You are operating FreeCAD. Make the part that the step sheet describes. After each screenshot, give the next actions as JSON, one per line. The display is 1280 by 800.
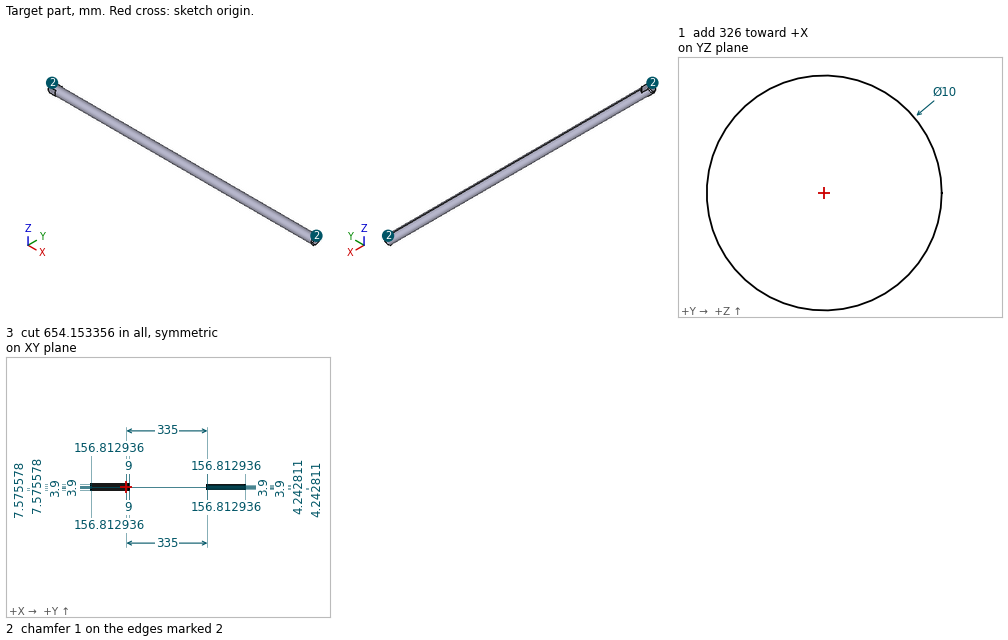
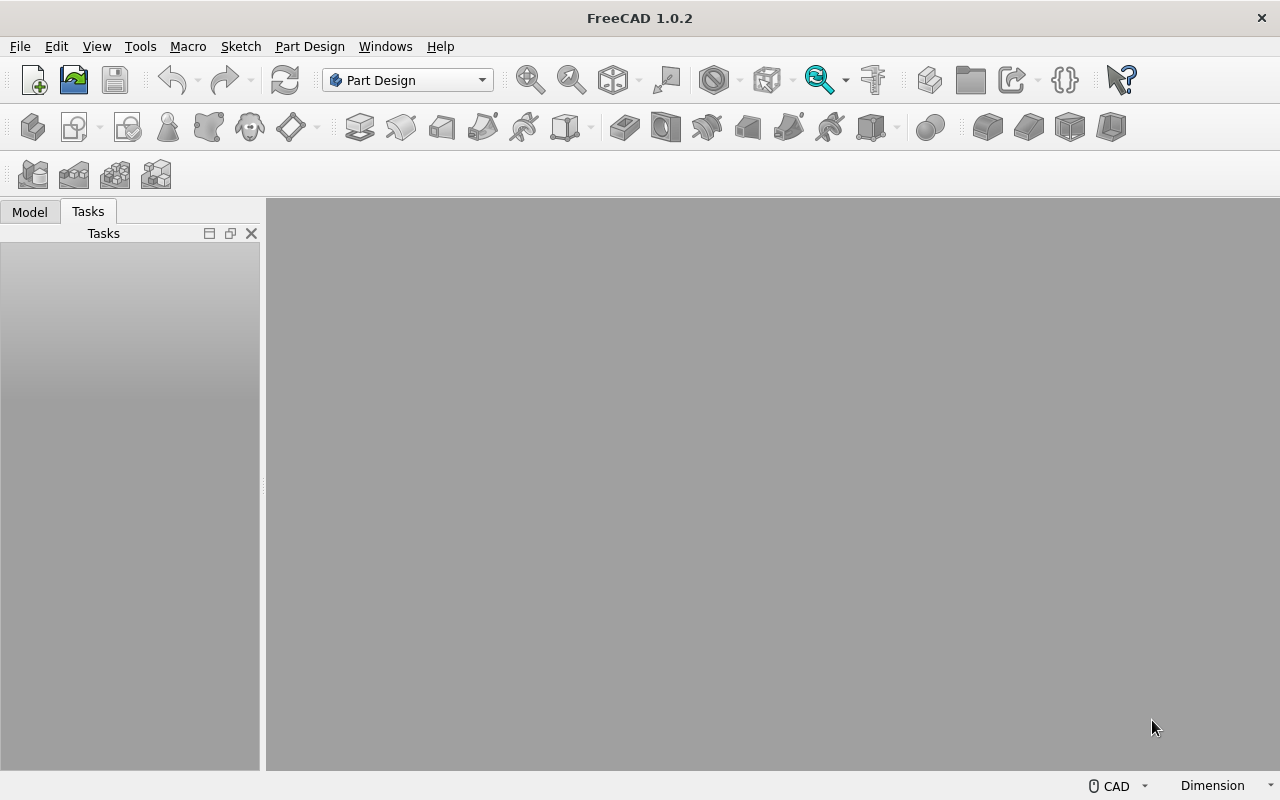
{"action": "left_click", "coordinate": [33, 80]}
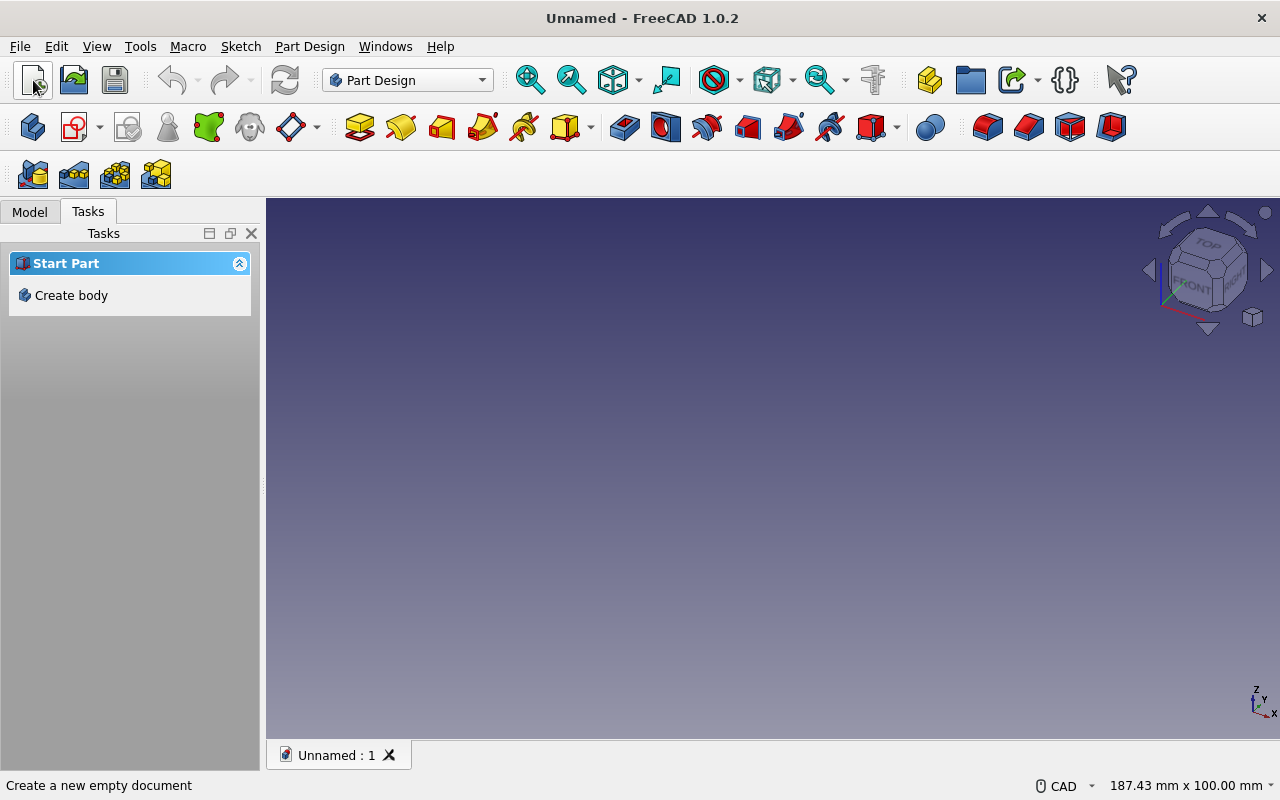
{"action": "left_click", "coordinate": [74, 128]}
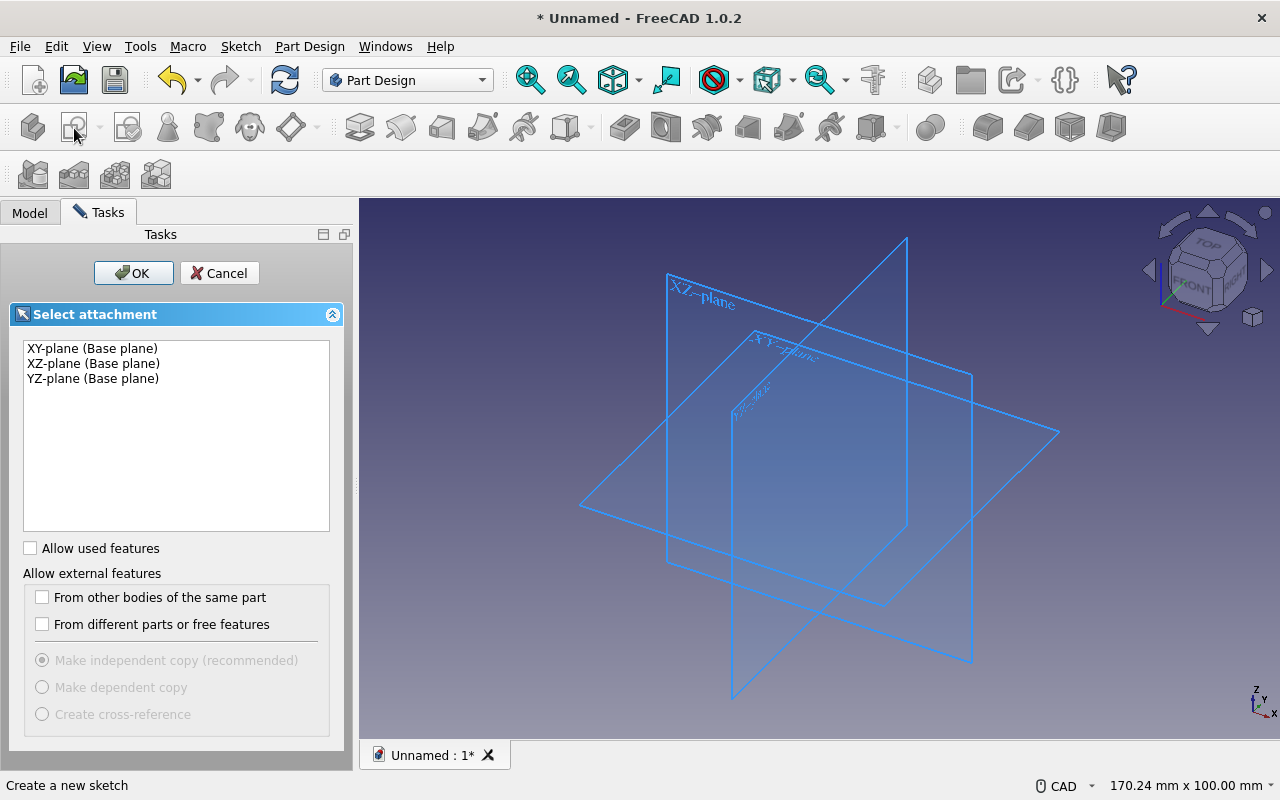
{"action": "left_click", "coordinate": [84, 378]}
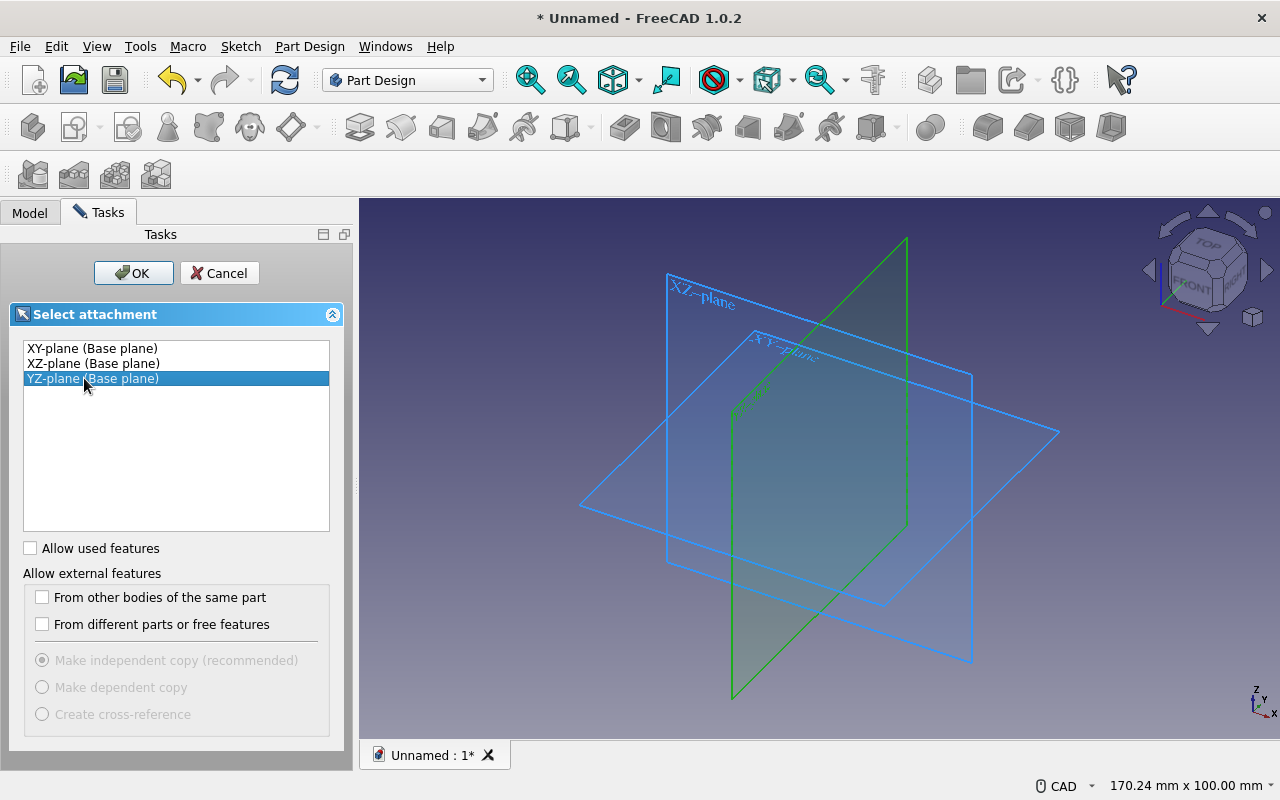
{"action": "left_click", "coordinate": [134, 273]}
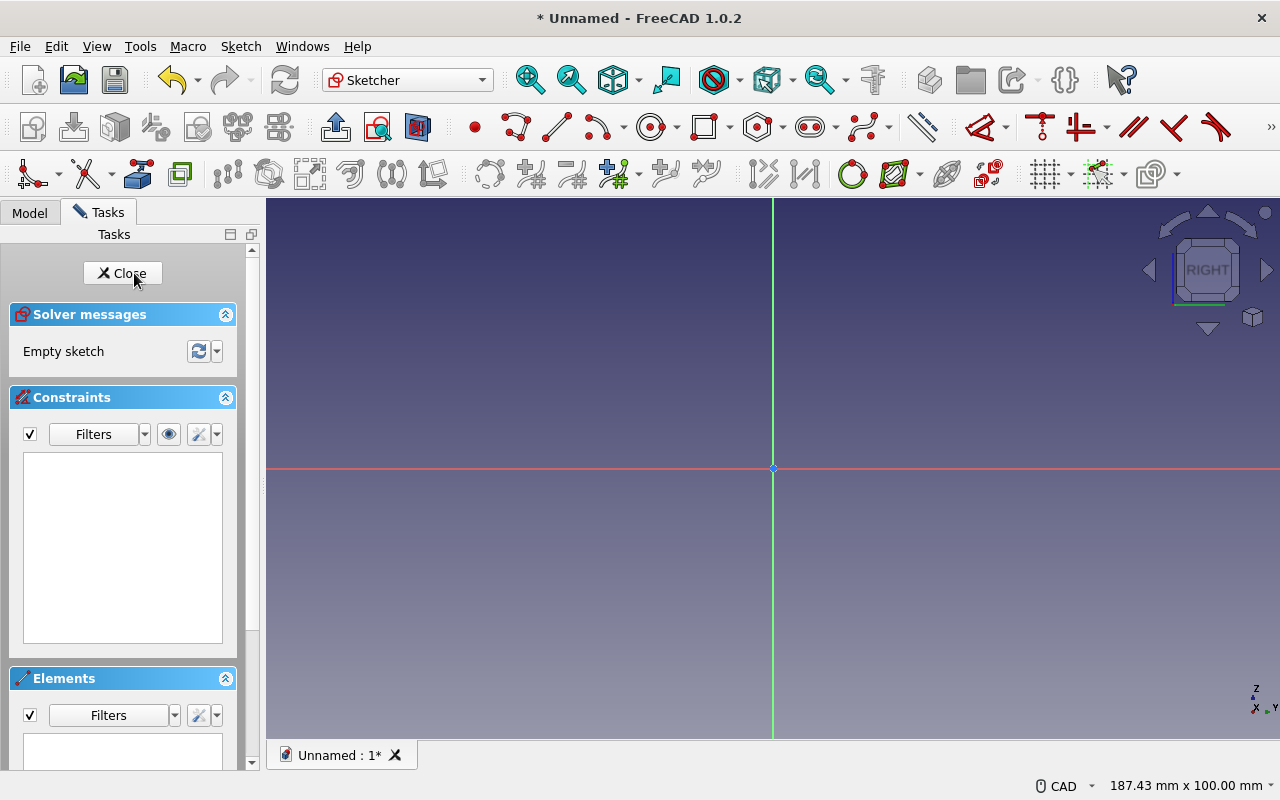
{"action": "scroll", "coordinate": [787, 468], "scroll_direction": "up", "scroll_amount": 9}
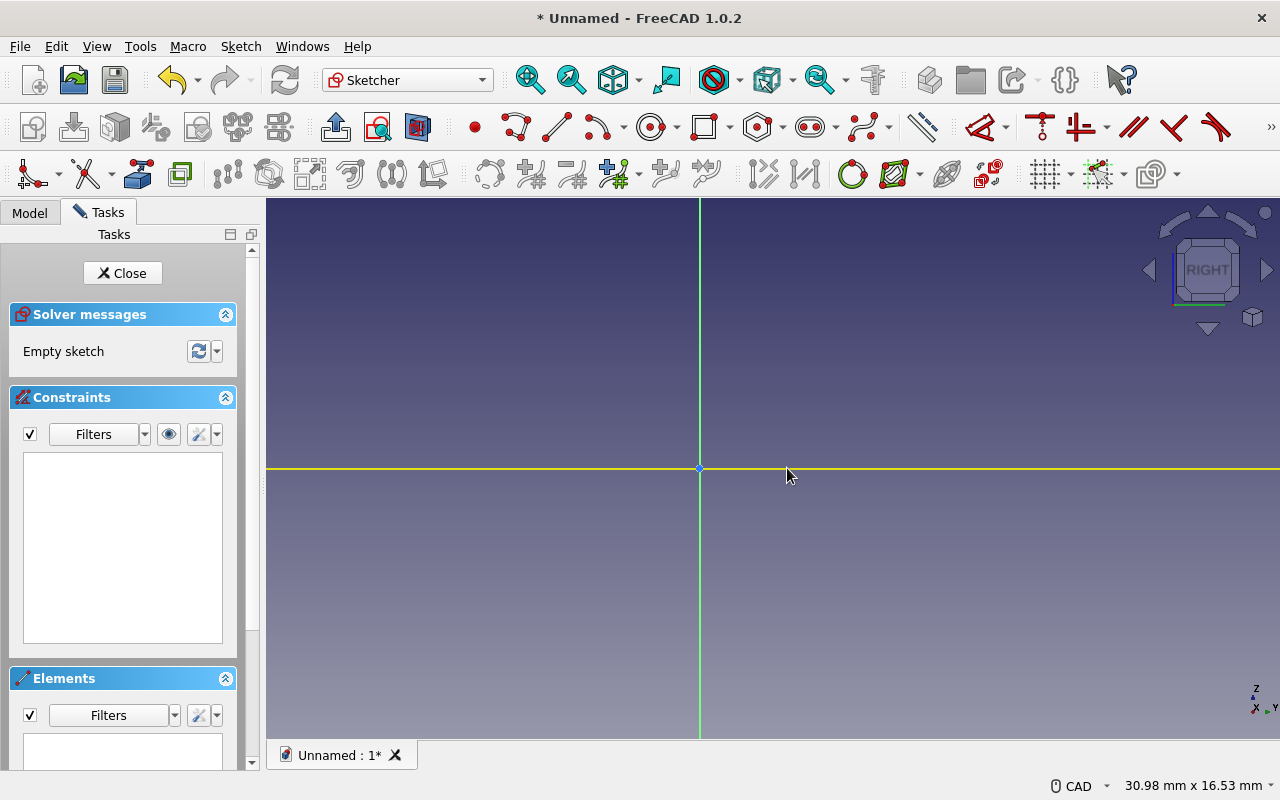
{"action": "key", "text": "g c"}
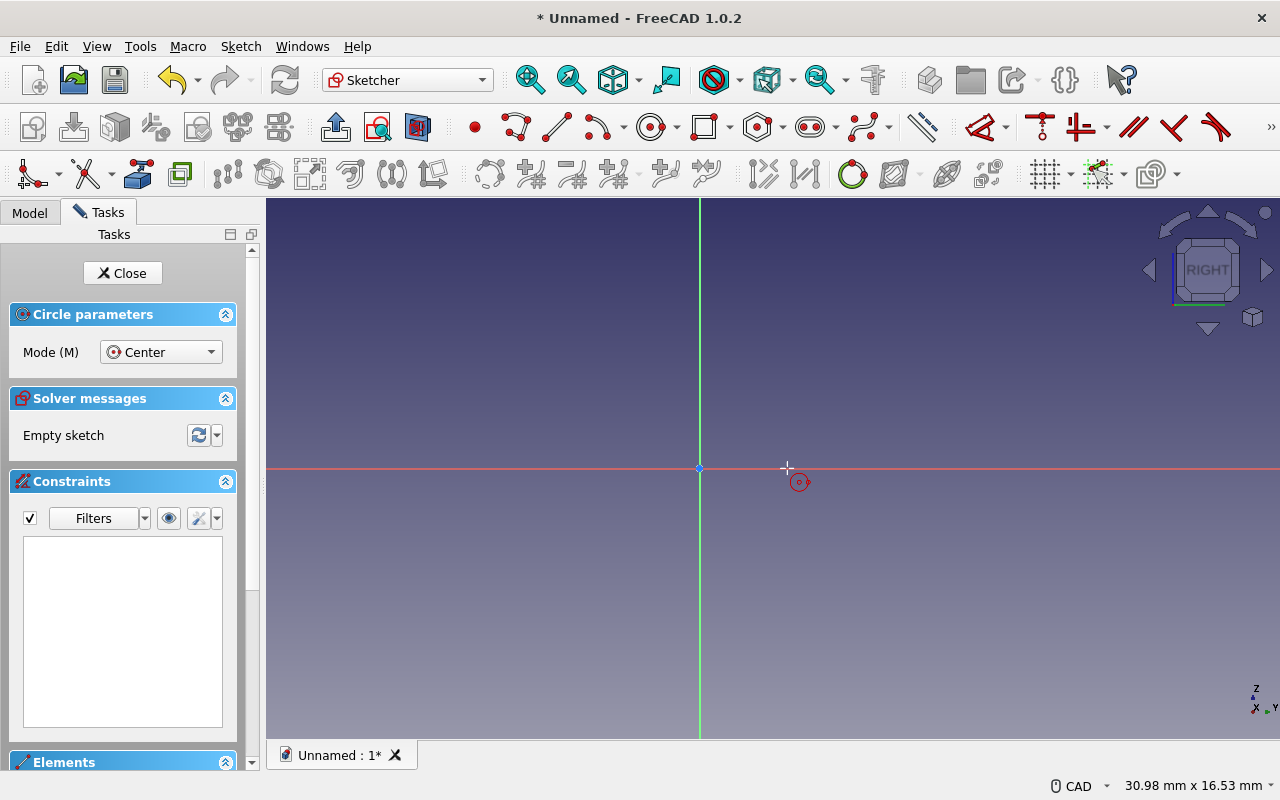
{"action": "left_click", "coordinate": [700, 468]}
{"action": "left_click", "coordinate": [815, 353]}
{"action": "key", "text": "Escape"}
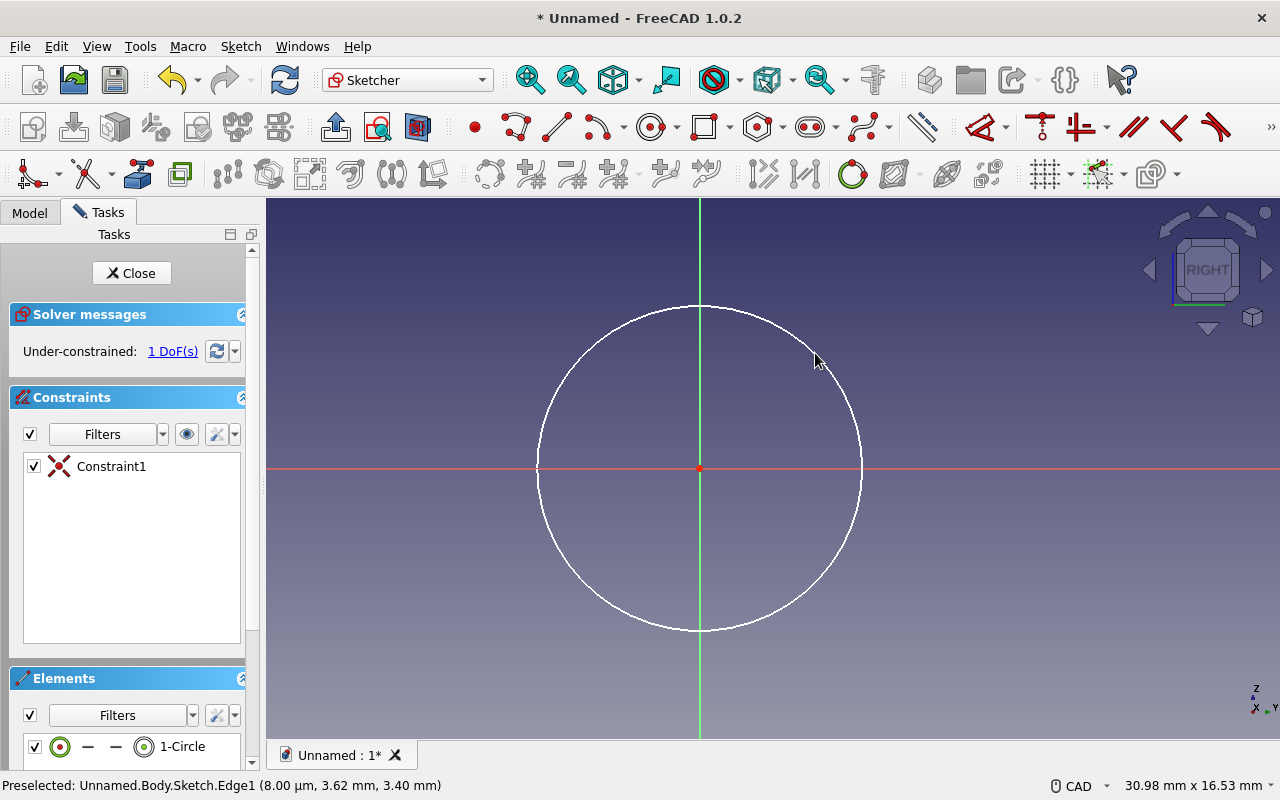
{"action": "left_click", "coordinate": [980, 128]}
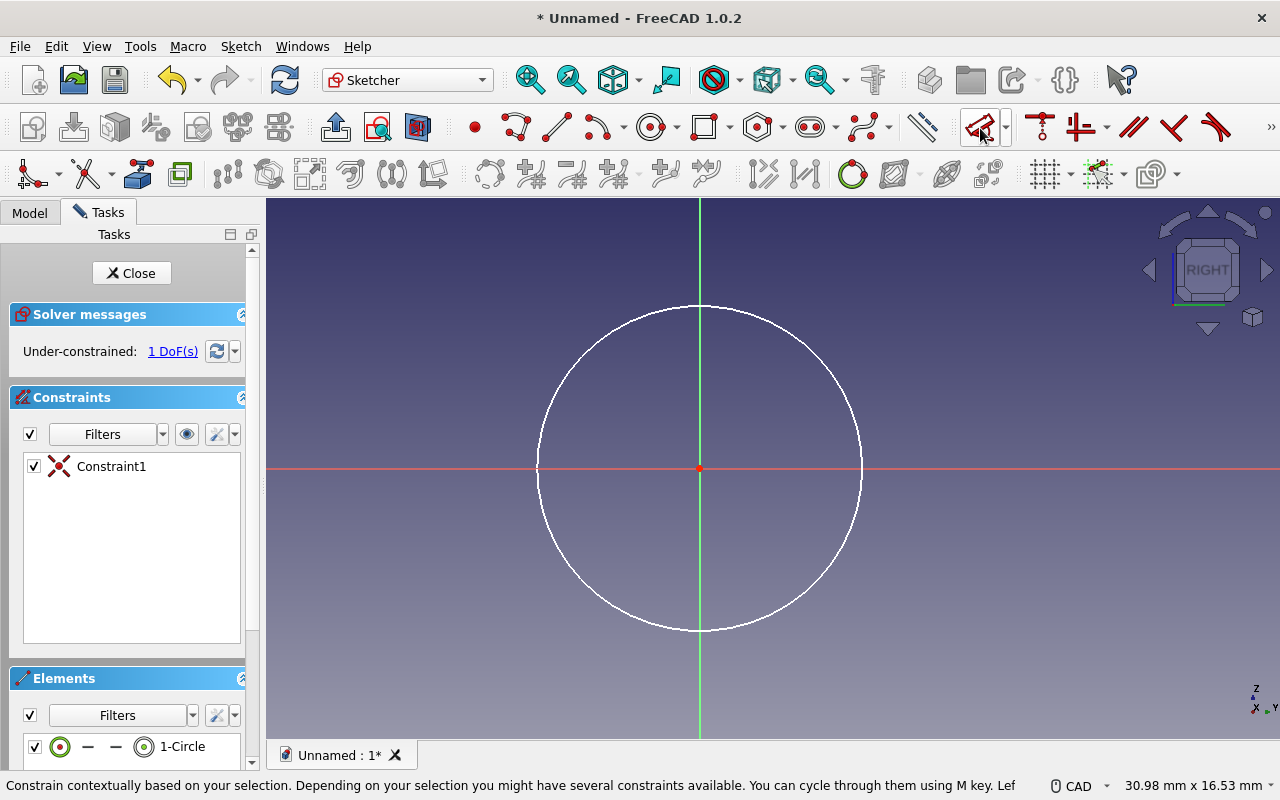
{"action": "left_click", "coordinate": [814, 353]}
{"action": "left_click", "coordinate": [837, 330]}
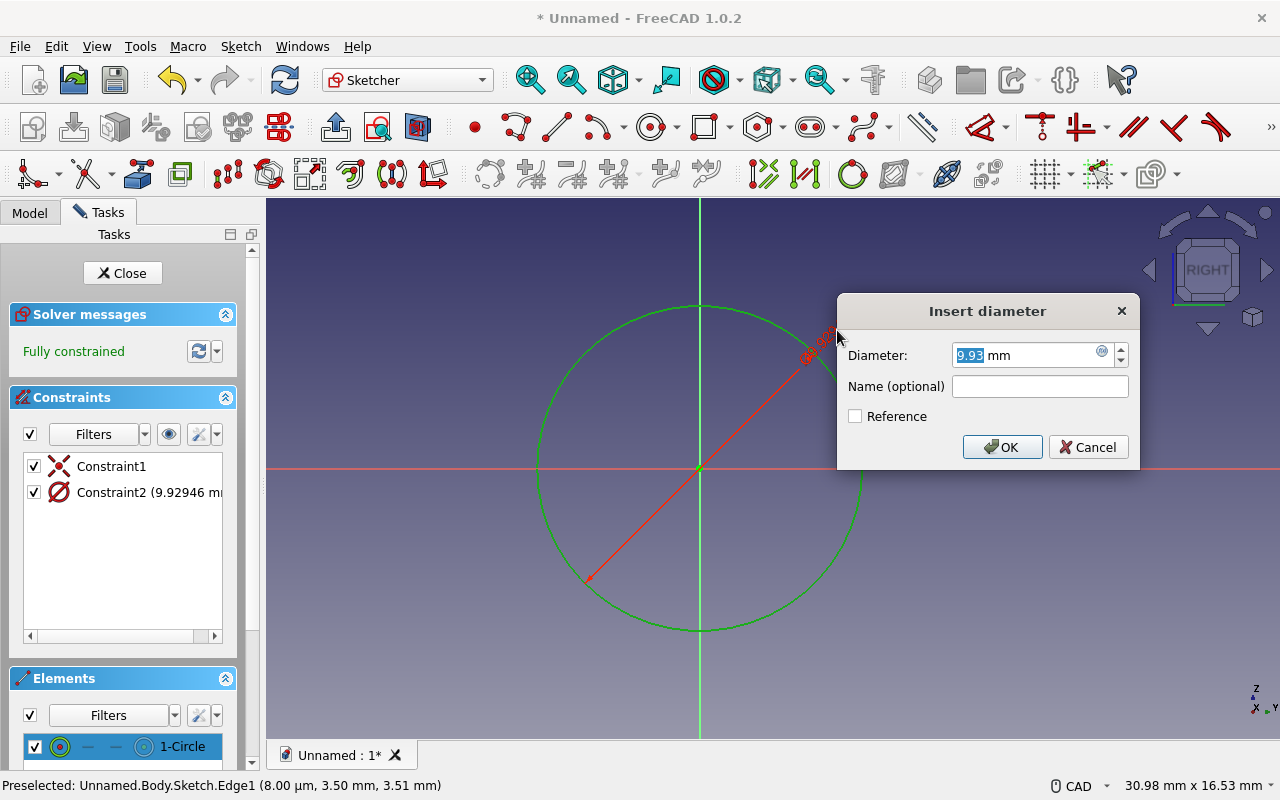
{"action": "type", "text": "10"}
{"action": "key", "text": "Return"}
{"action": "key", "text": "Escape"}